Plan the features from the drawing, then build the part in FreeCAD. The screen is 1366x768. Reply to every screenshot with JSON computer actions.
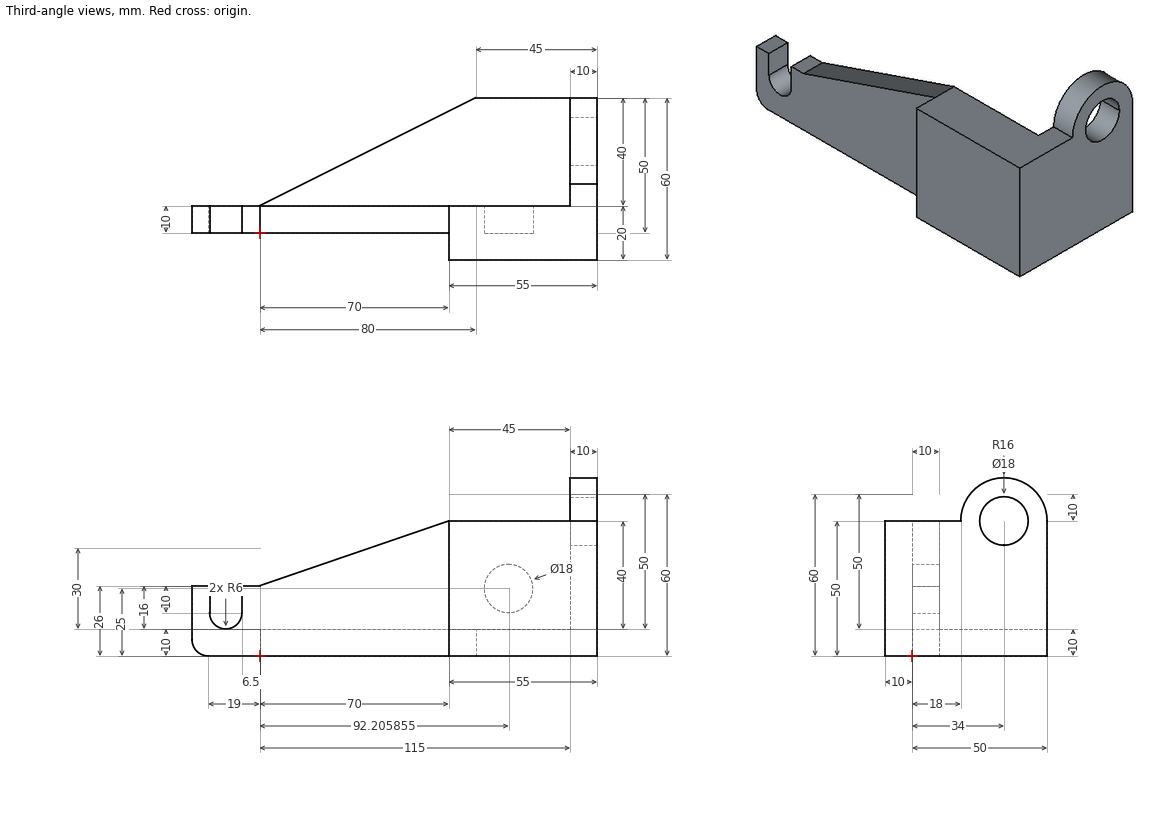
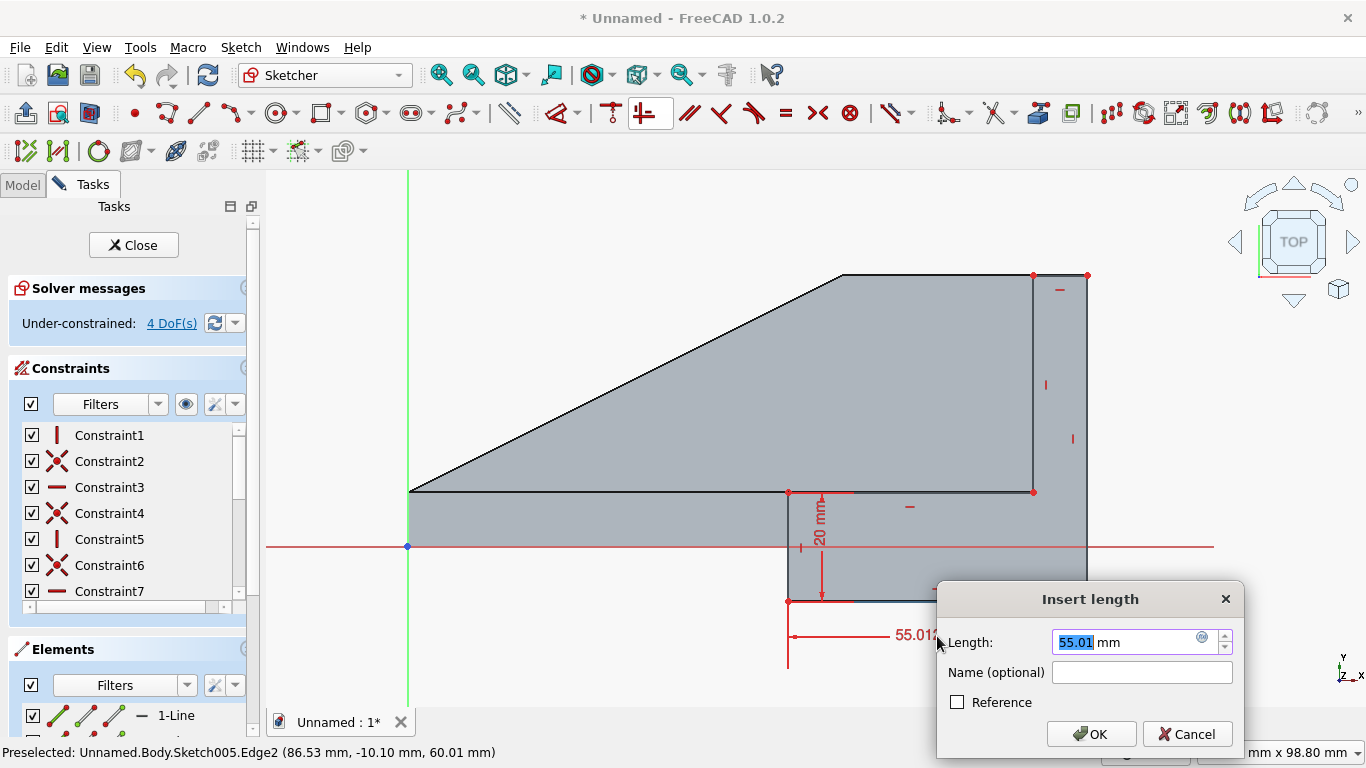
{"action": "type", "text": "55"}
{"action": "key", "text": "Return"}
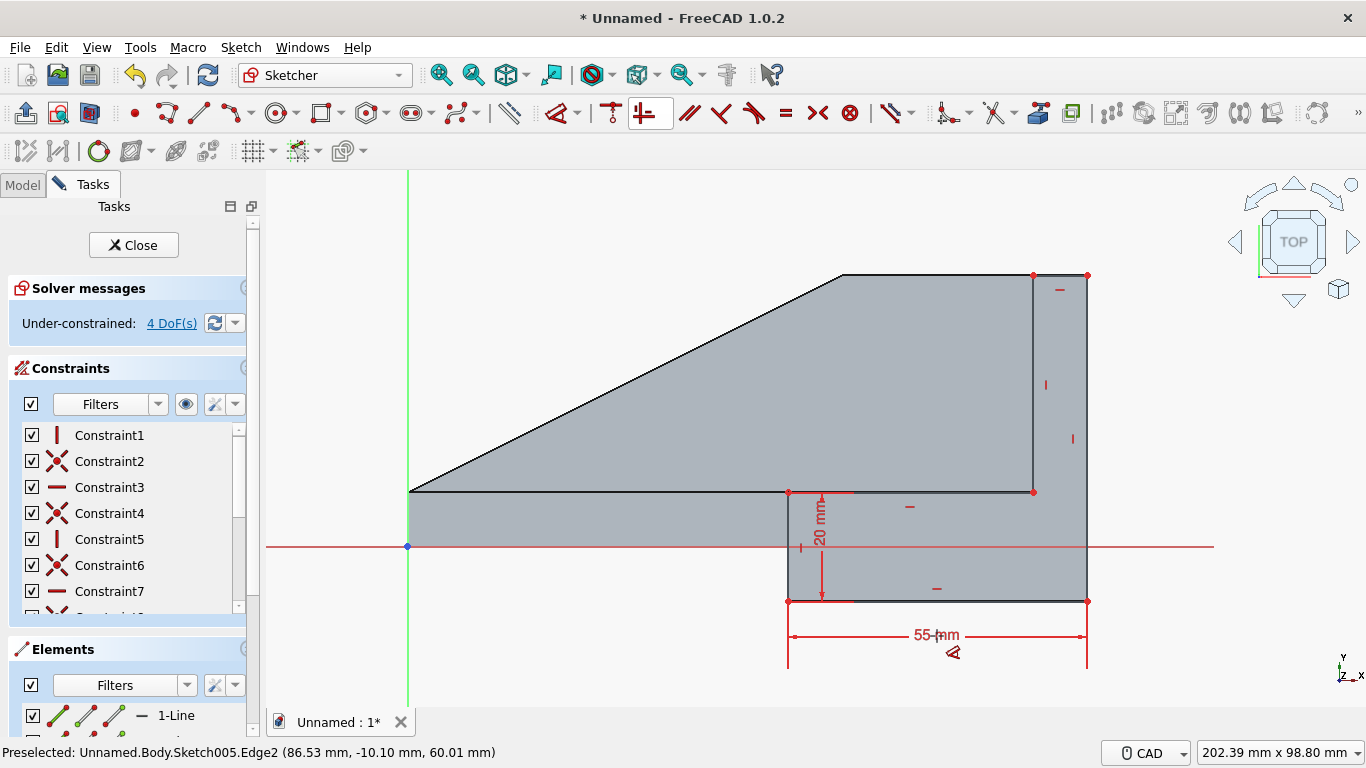
{"action": "left_click", "coordinate": [1087, 504]}
{"action": "left_click", "coordinate": [1121, 439]}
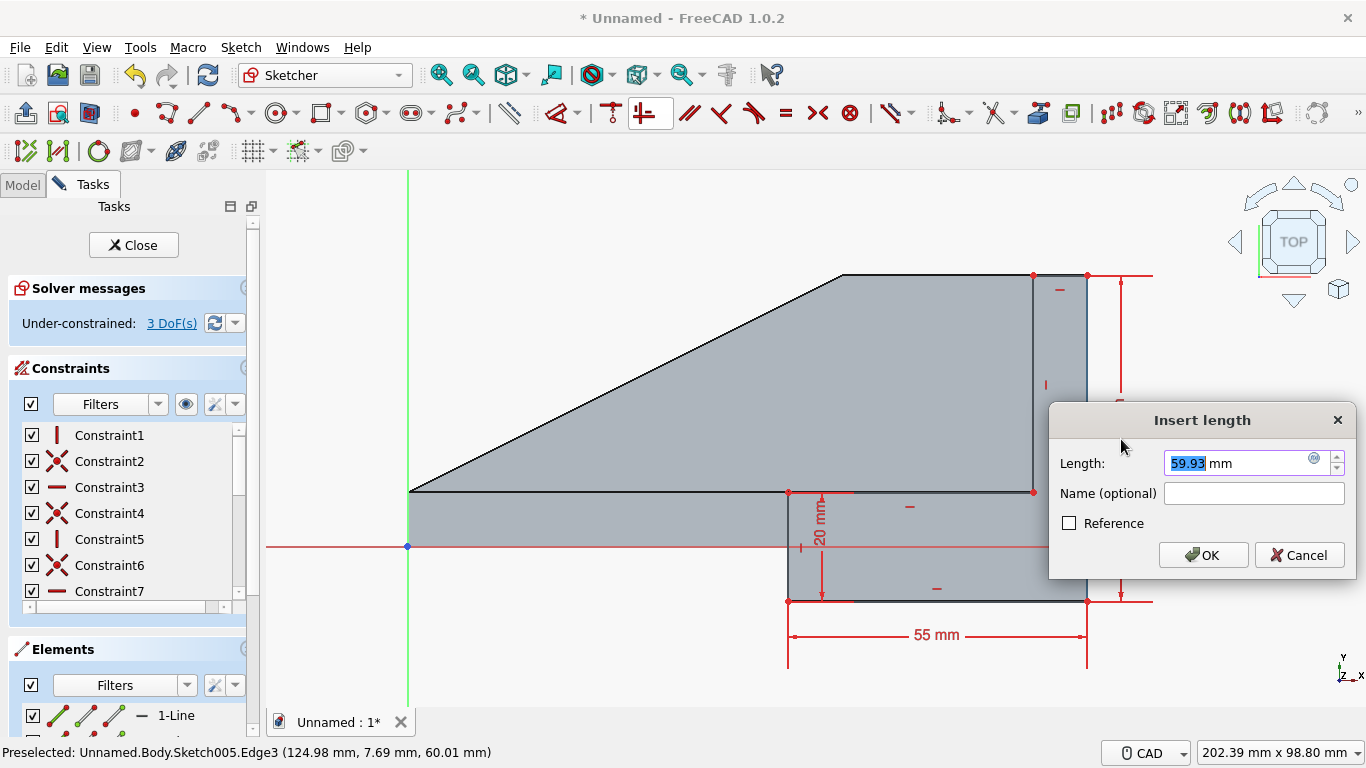
{"action": "type", "text": "60"}
{"action": "key", "text": "Return"}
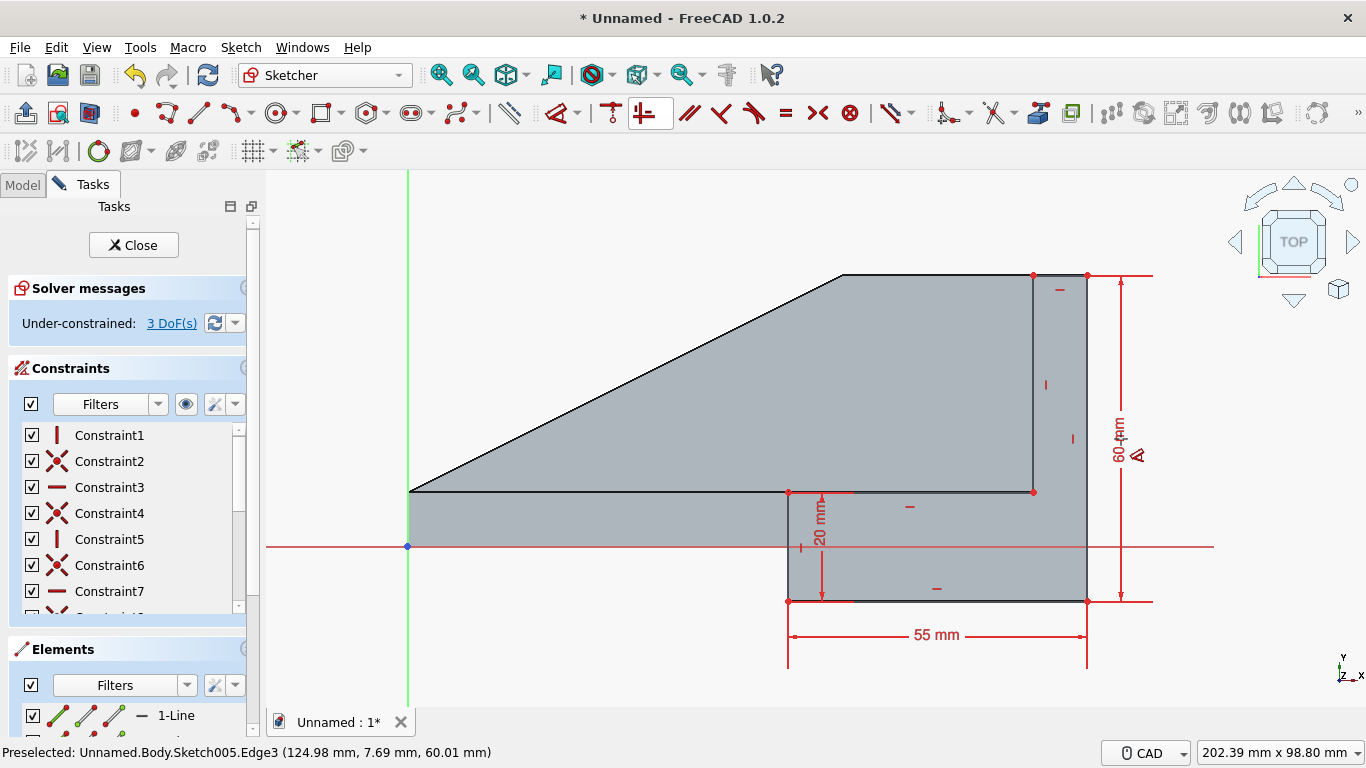
{"action": "left_click", "coordinate": [1071, 276]}
{"action": "left_click", "coordinate": [1060, 242]}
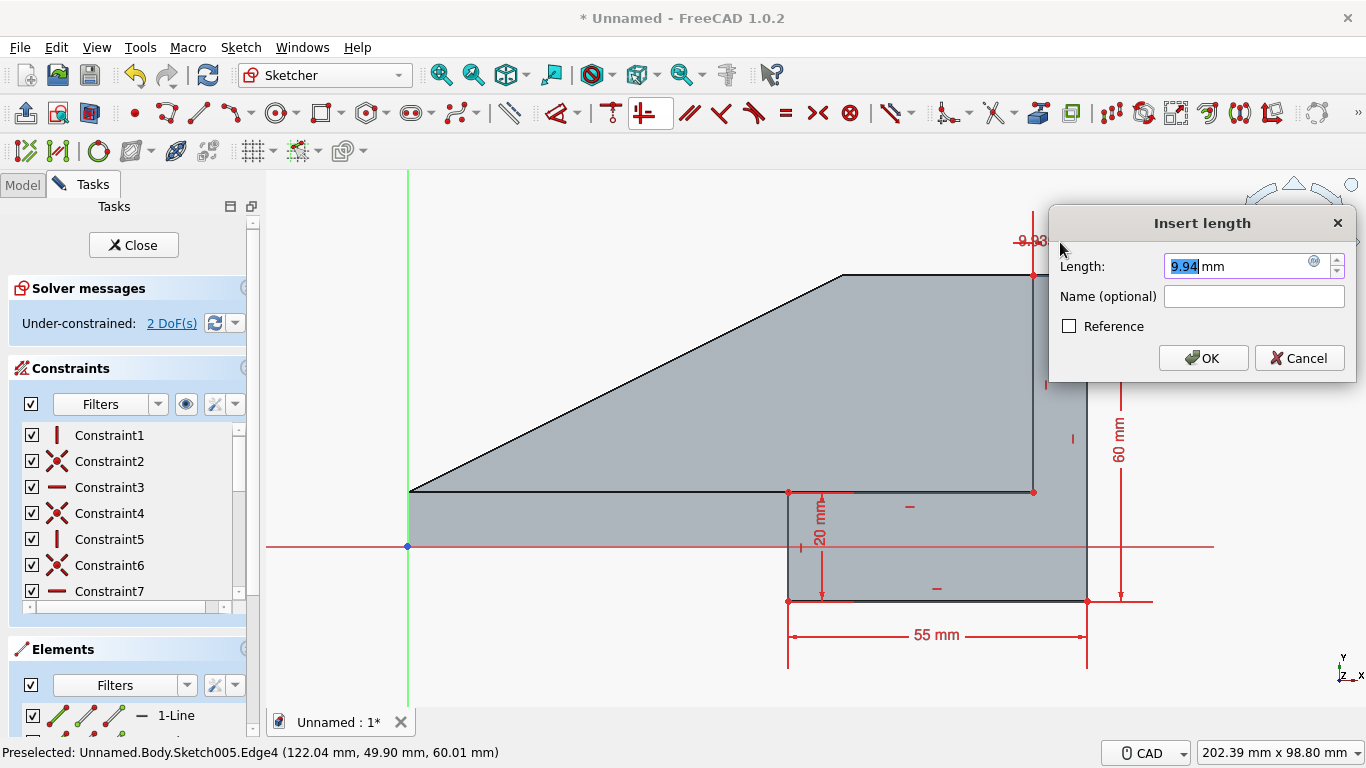
{"action": "type", "text": "10"}
{"action": "key", "text": "Return"}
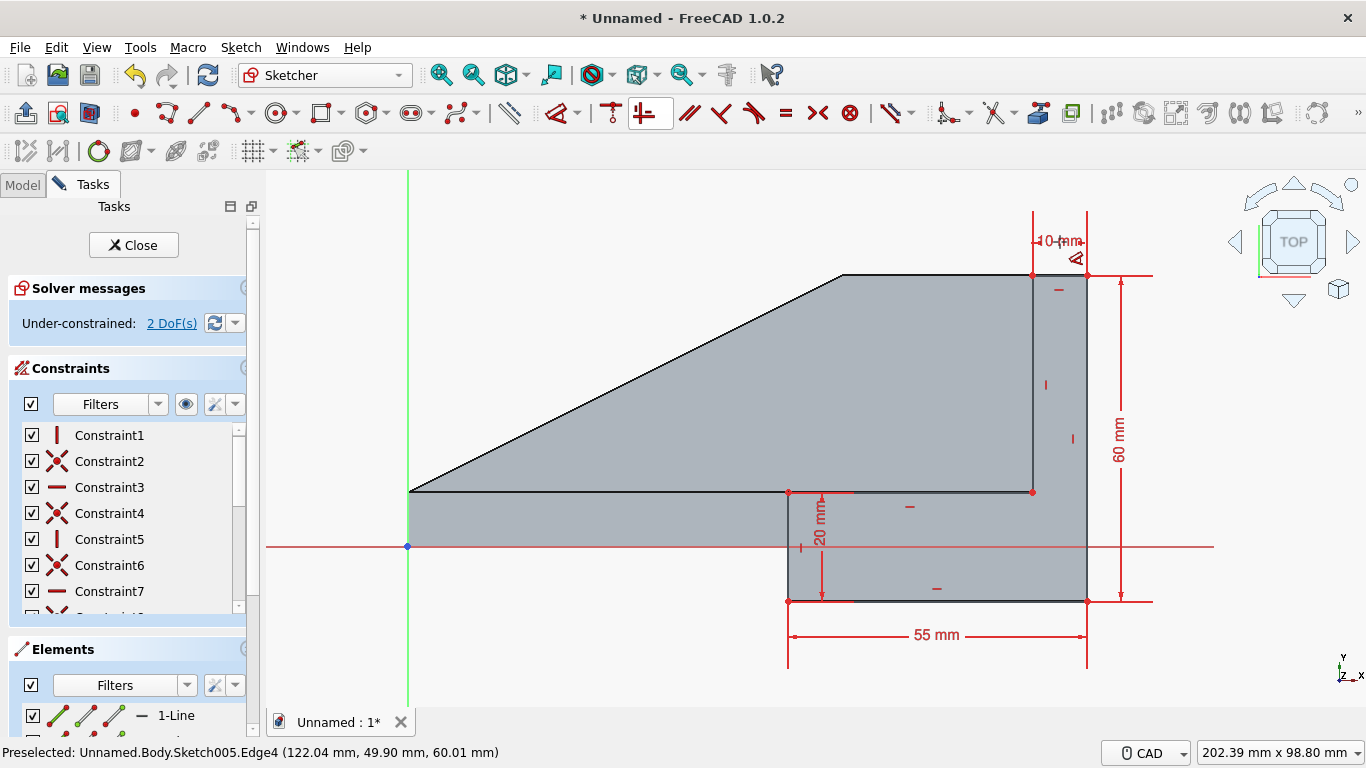
{"action": "left_click", "coordinate": [788, 493]}
{"action": "left_click", "coordinate": [598, 581]}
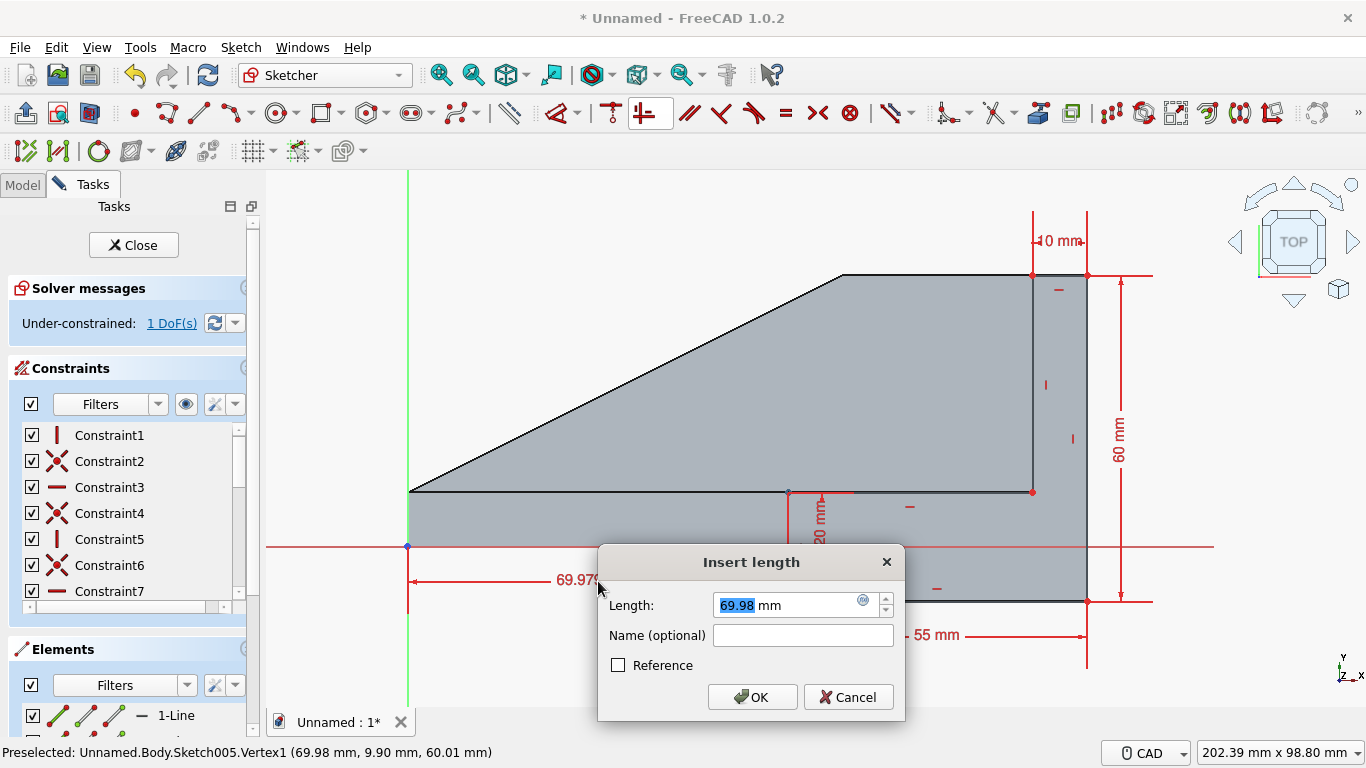
{"action": "type", "text": "70"}
{"action": "key", "text": "Return"}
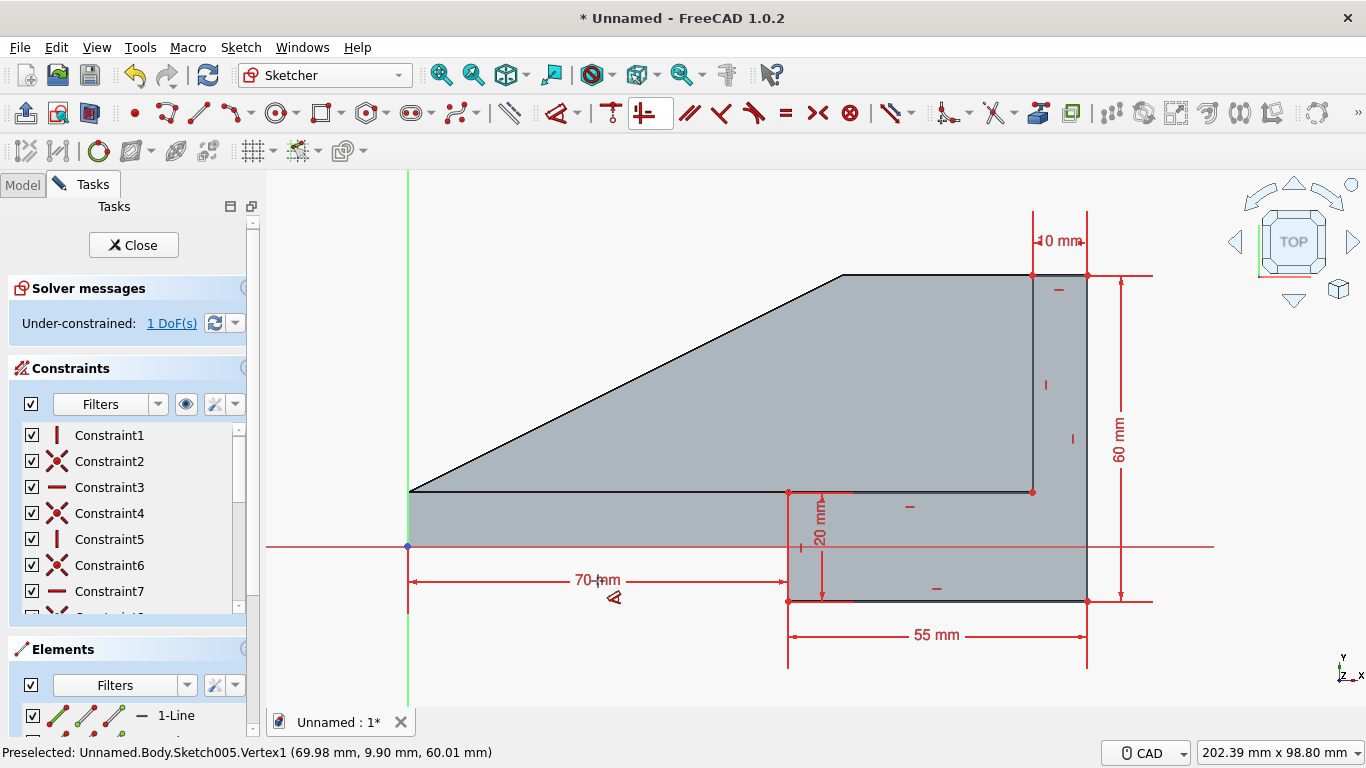
{"action": "left_click", "coordinate": [788, 493]}
{"action": "left_click", "coordinate": [374, 520]}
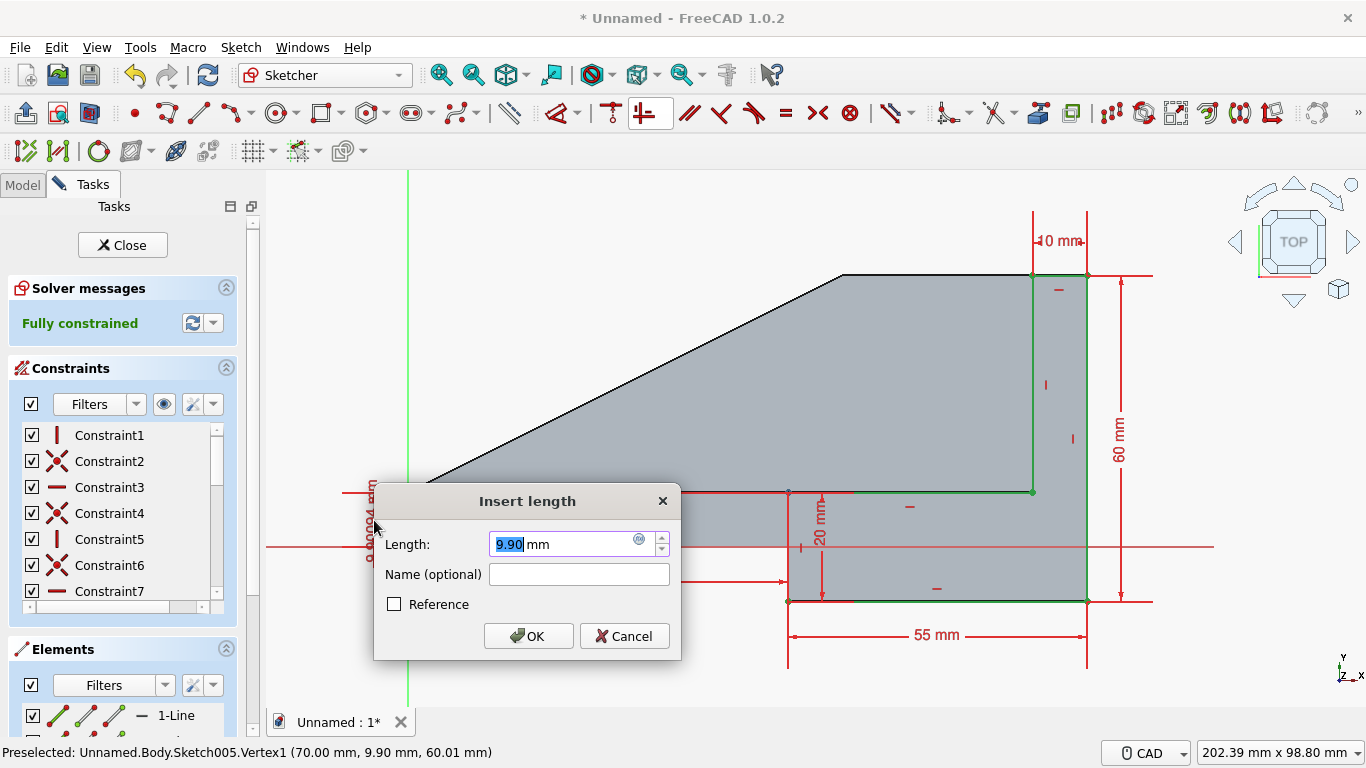
{"action": "type", "text": "10"}
{"action": "key", "text": "Return"}
{"action": "key", "text": "Escape"}